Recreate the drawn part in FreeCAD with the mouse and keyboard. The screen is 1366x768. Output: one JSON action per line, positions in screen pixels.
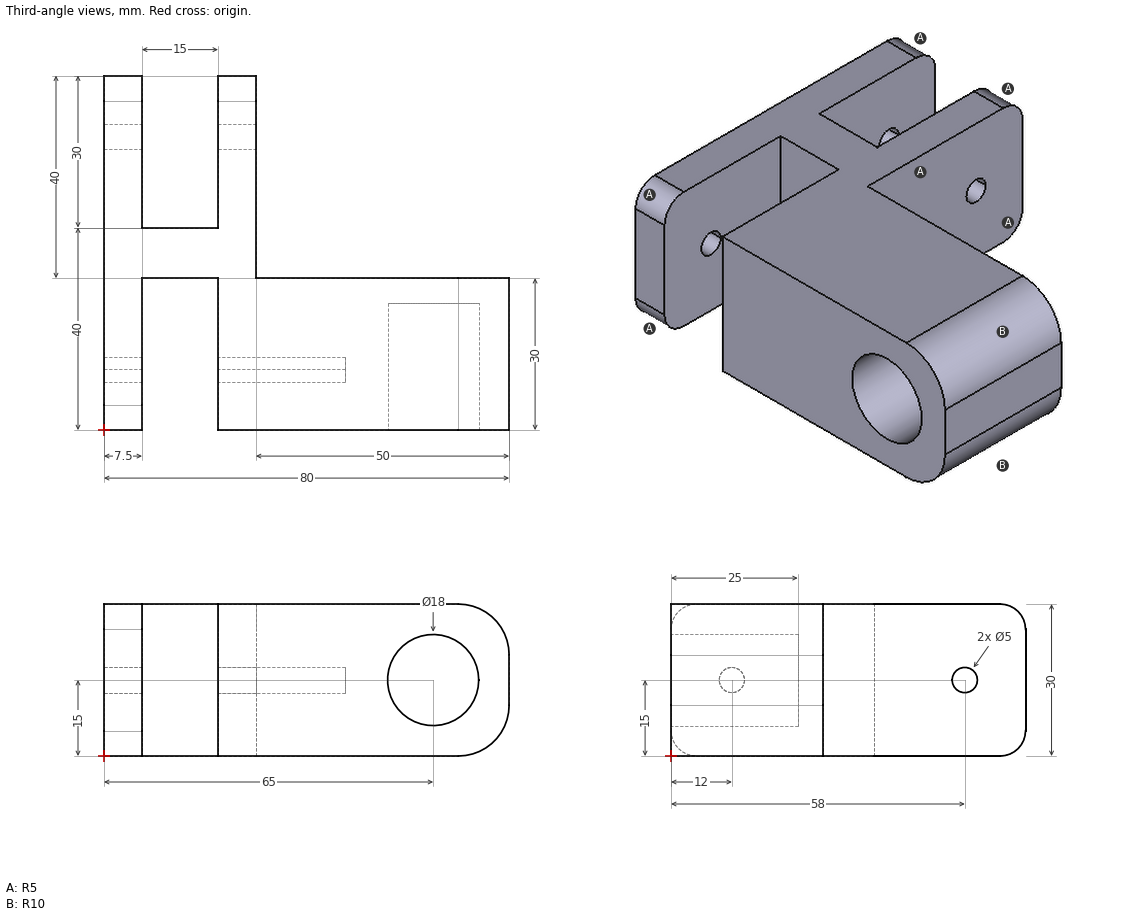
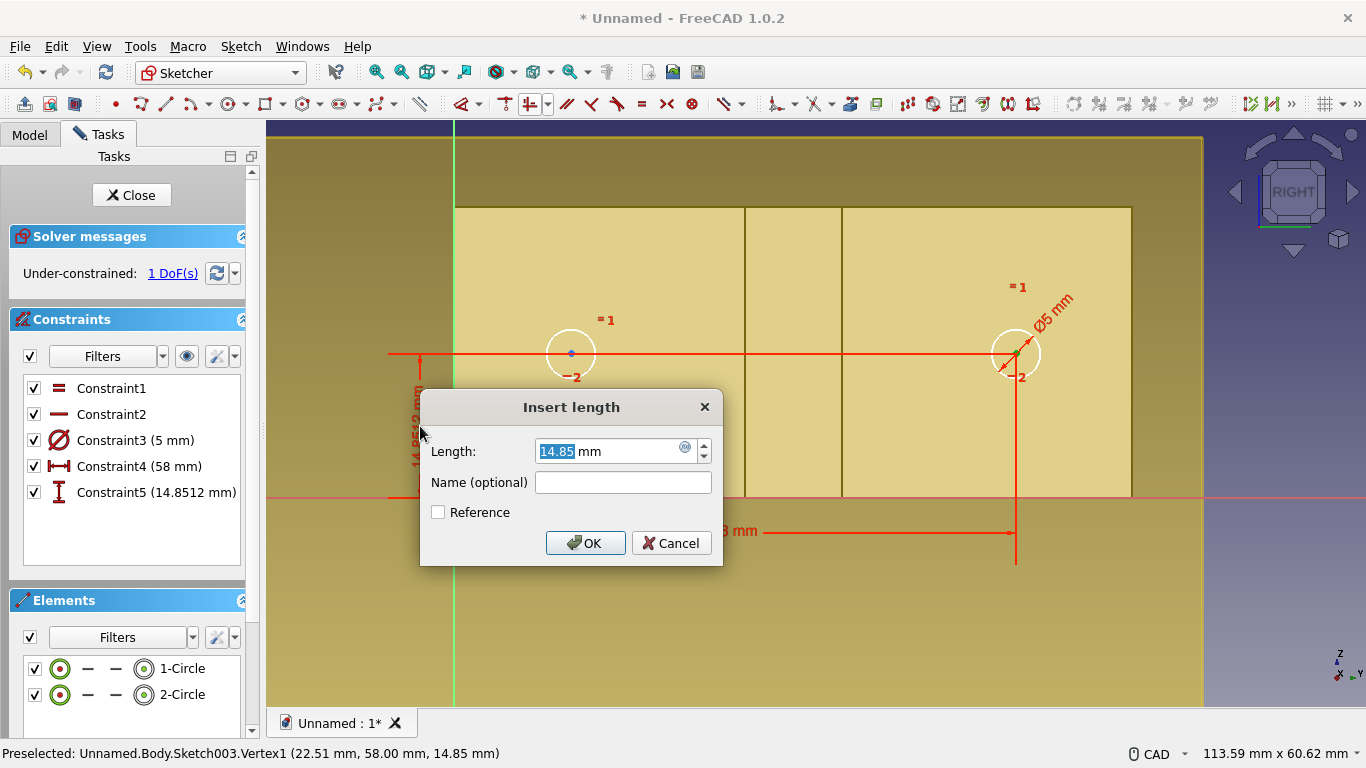
{"action": "type", "text": "15"}
{"action": "key", "text": "Return"}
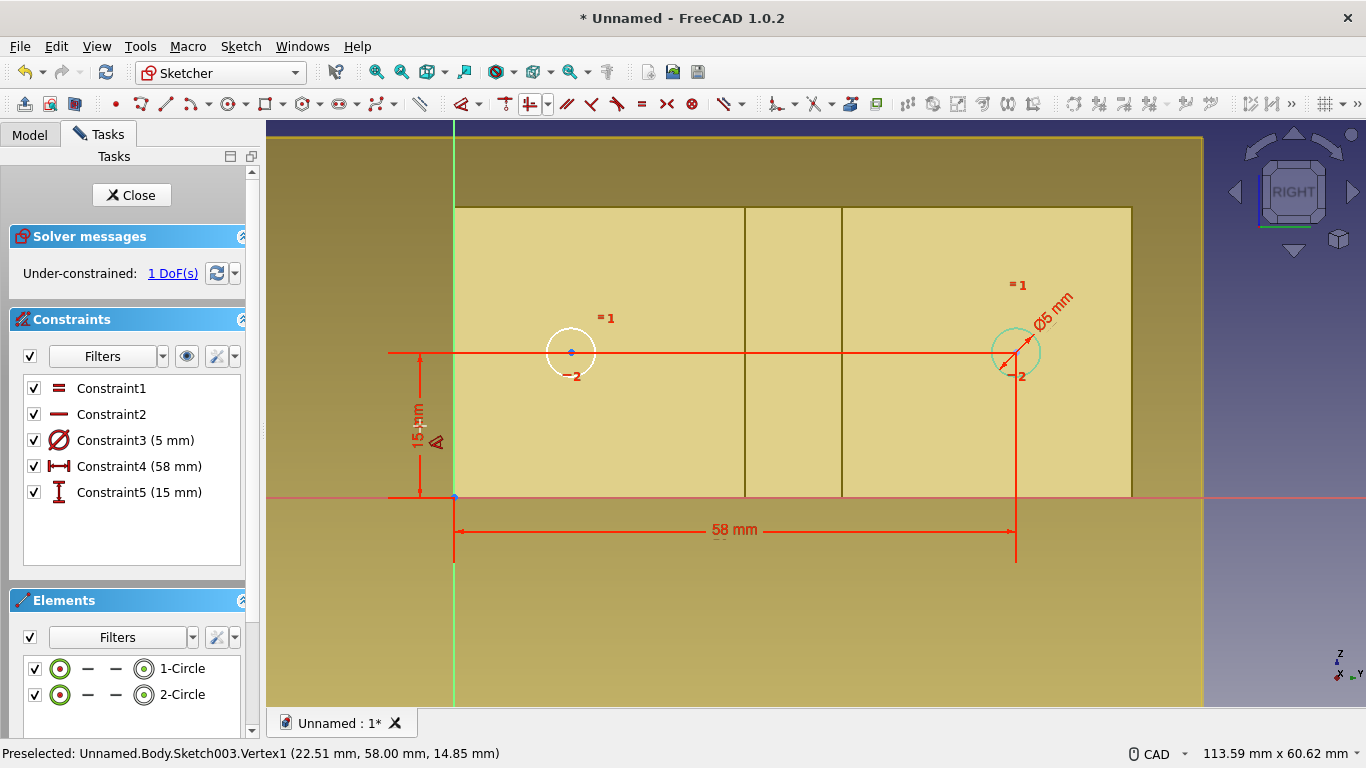
{"action": "left_click", "coordinate": [571, 353]}
{"action": "left_click", "coordinate": [513, 532]}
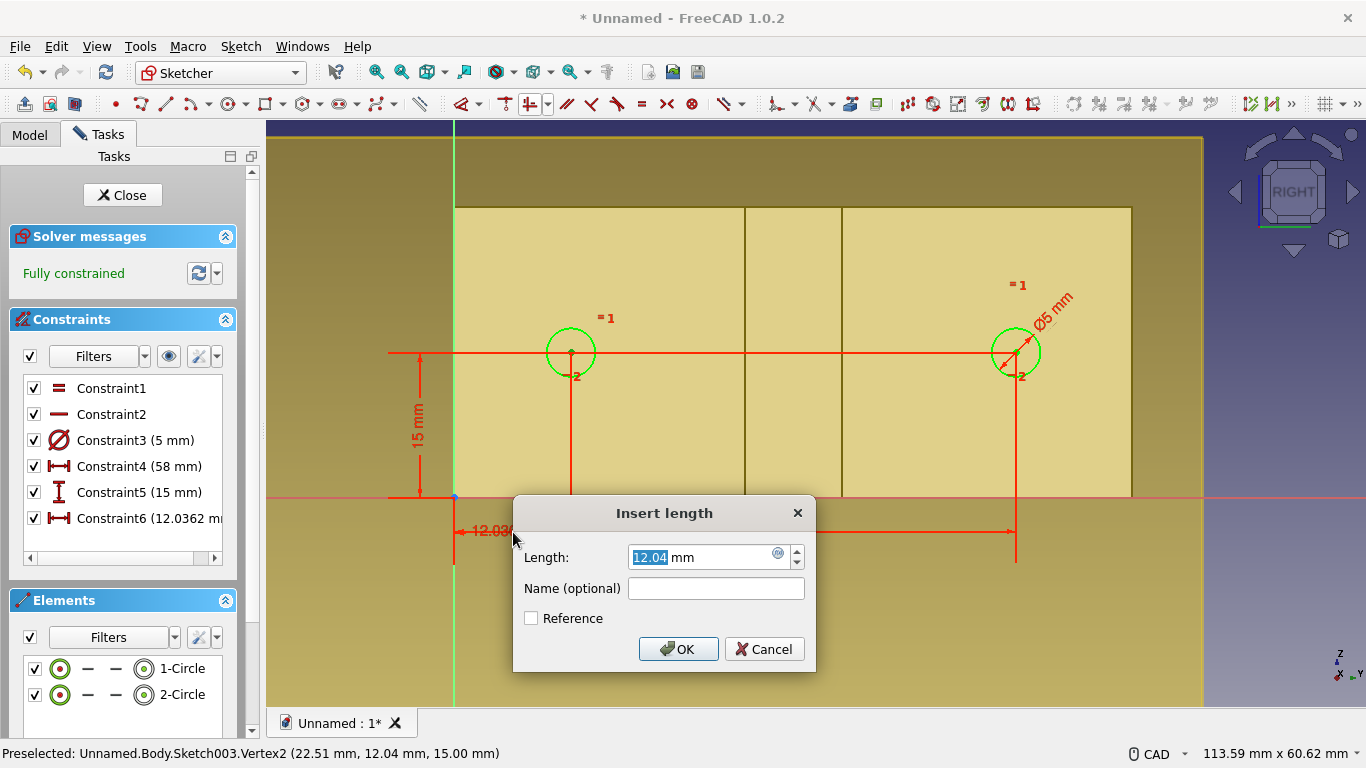
{"action": "type", "text": "12"}
{"action": "key", "text": "Return"}
{"action": "key", "text": "Escape"}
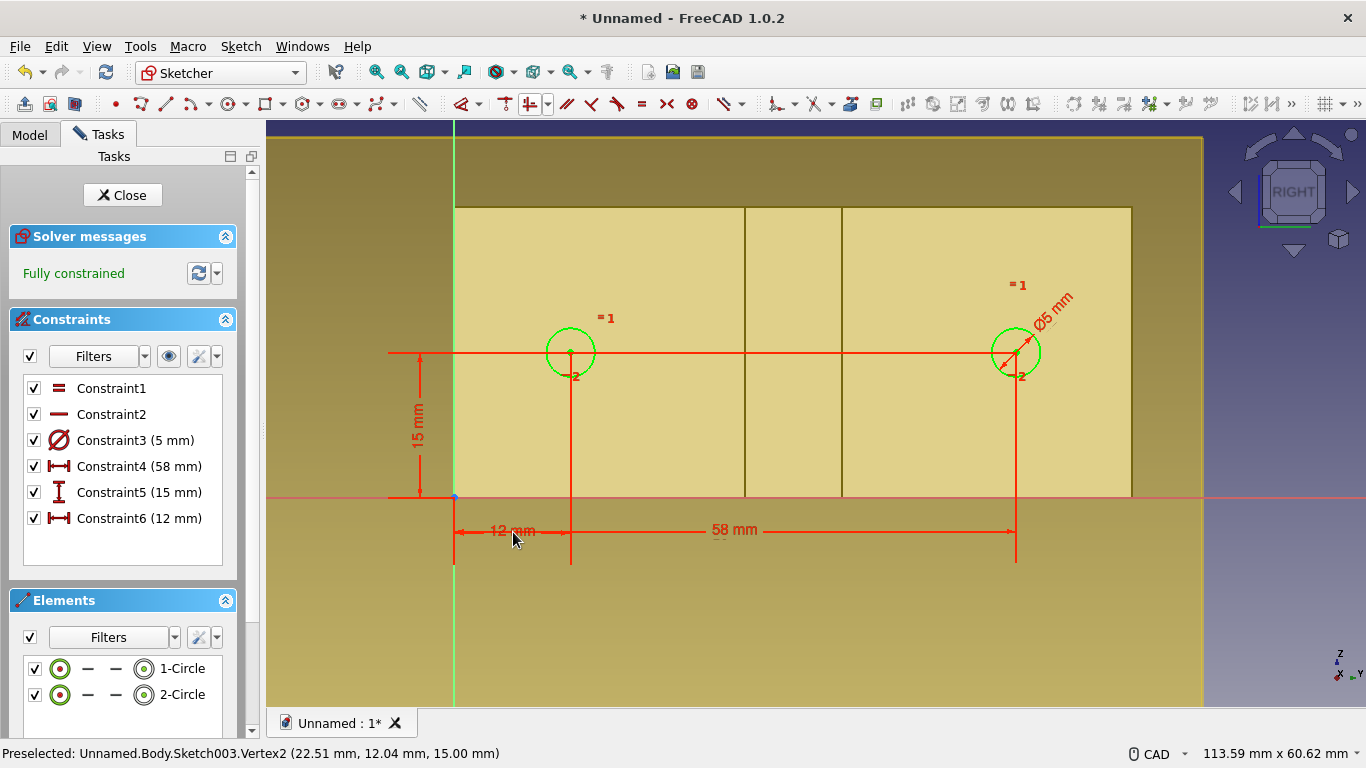
{"action": "left_click", "coordinate": [123, 195]}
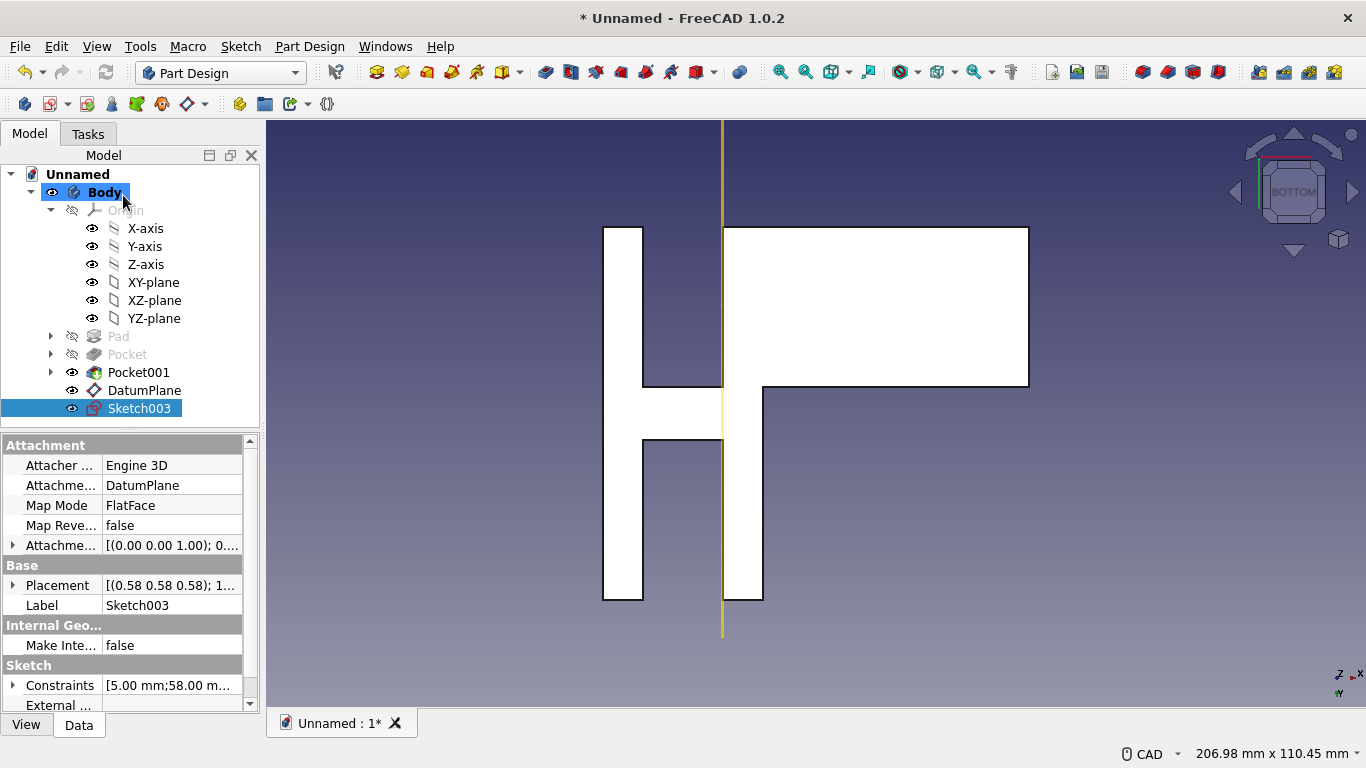
{"action": "left_click", "coordinate": [546, 72]}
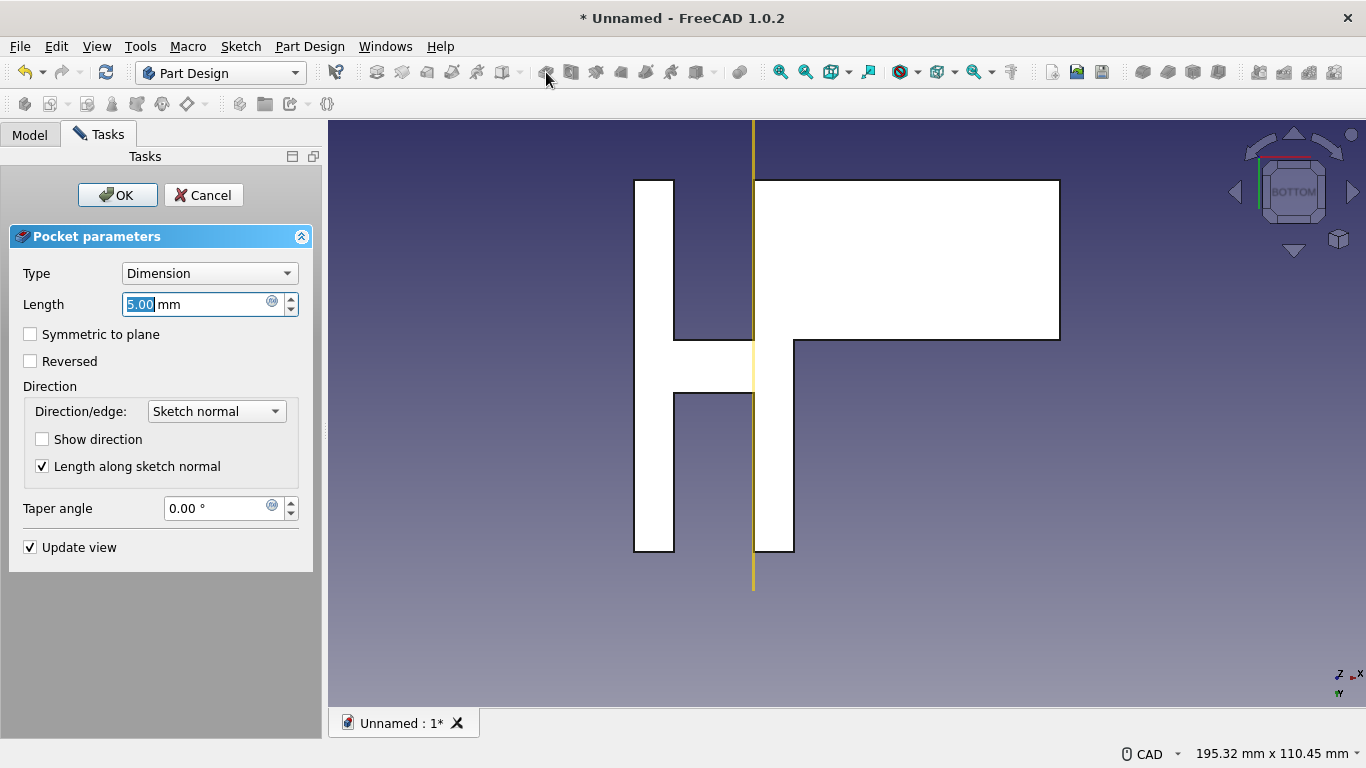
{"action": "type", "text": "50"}
{"action": "key", "text": "Tab"}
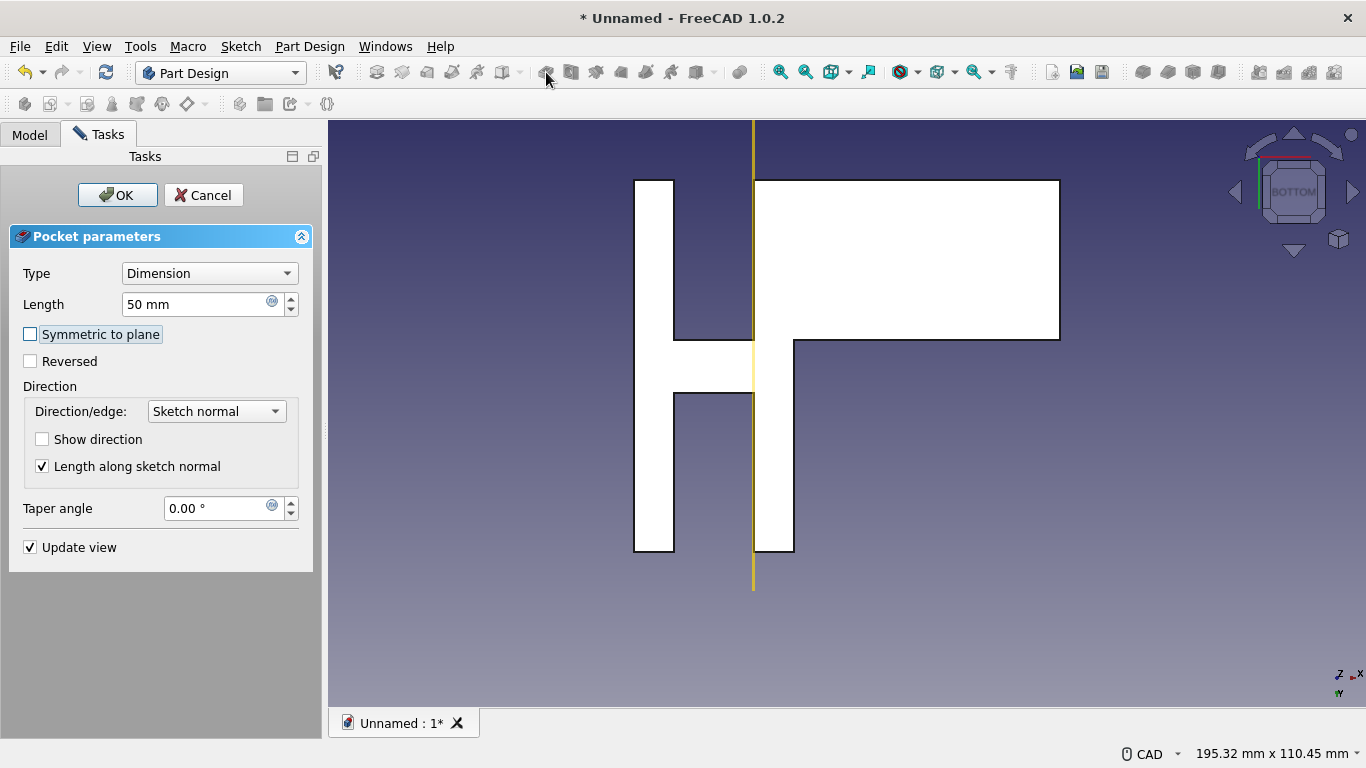
{"action": "left_click", "coordinate": [31, 334]}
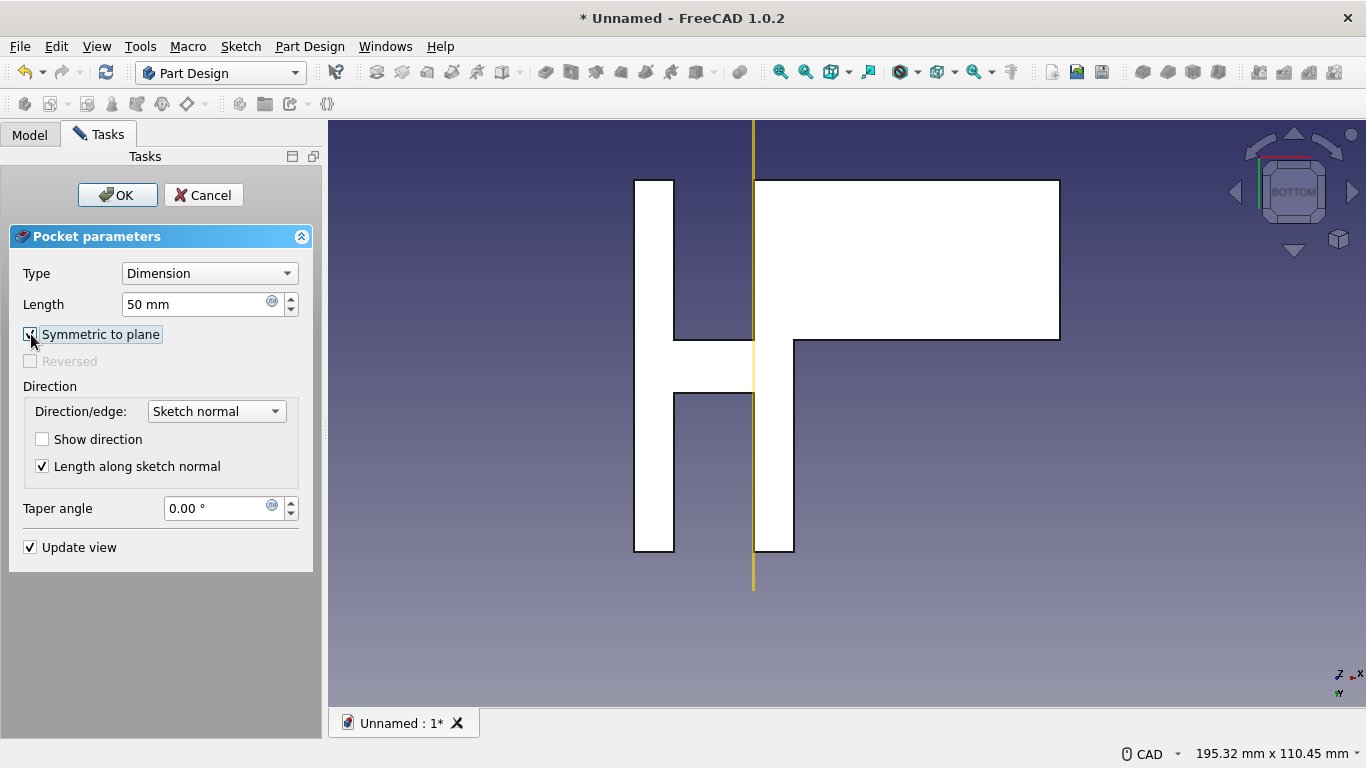
{"action": "left_click", "coordinate": [118, 195]}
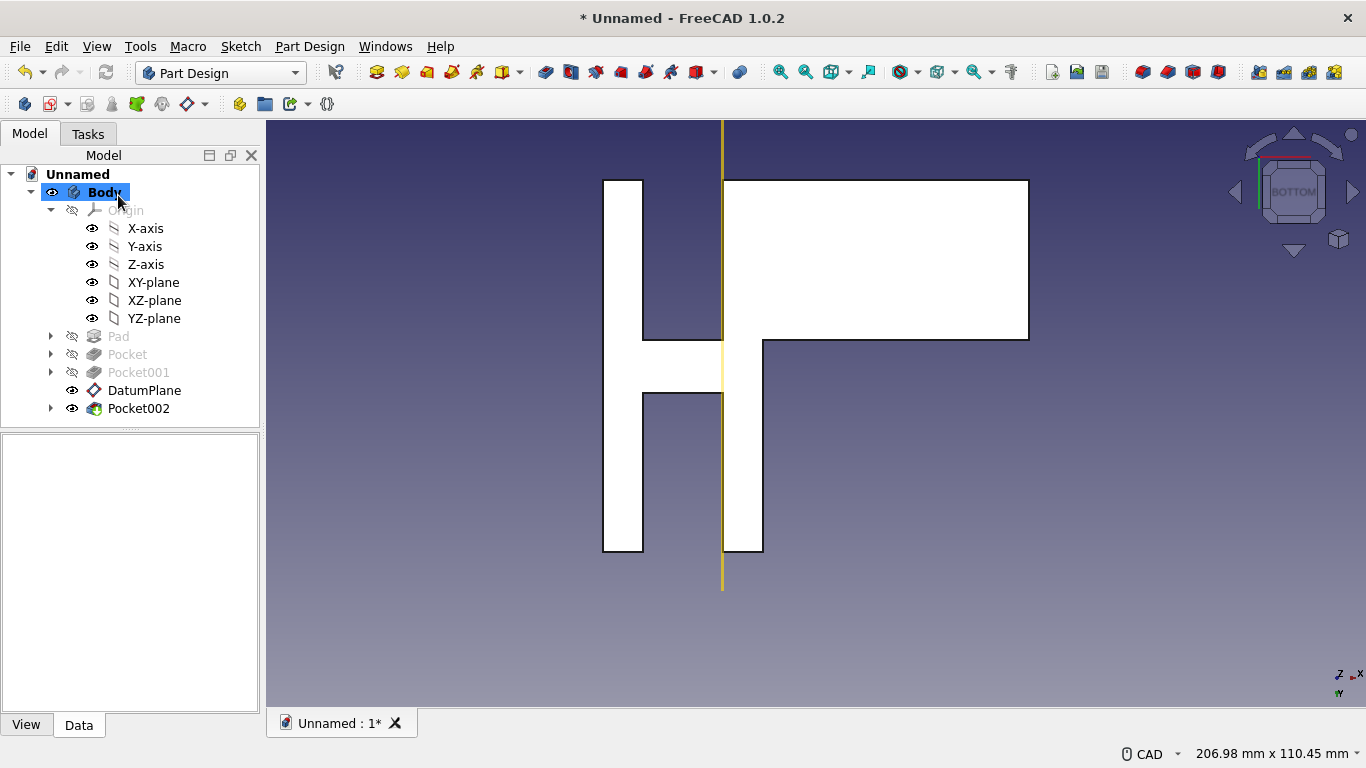
{"action": "left_click", "coordinate": [117, 390]}
{"action": "key", "text": "space"}